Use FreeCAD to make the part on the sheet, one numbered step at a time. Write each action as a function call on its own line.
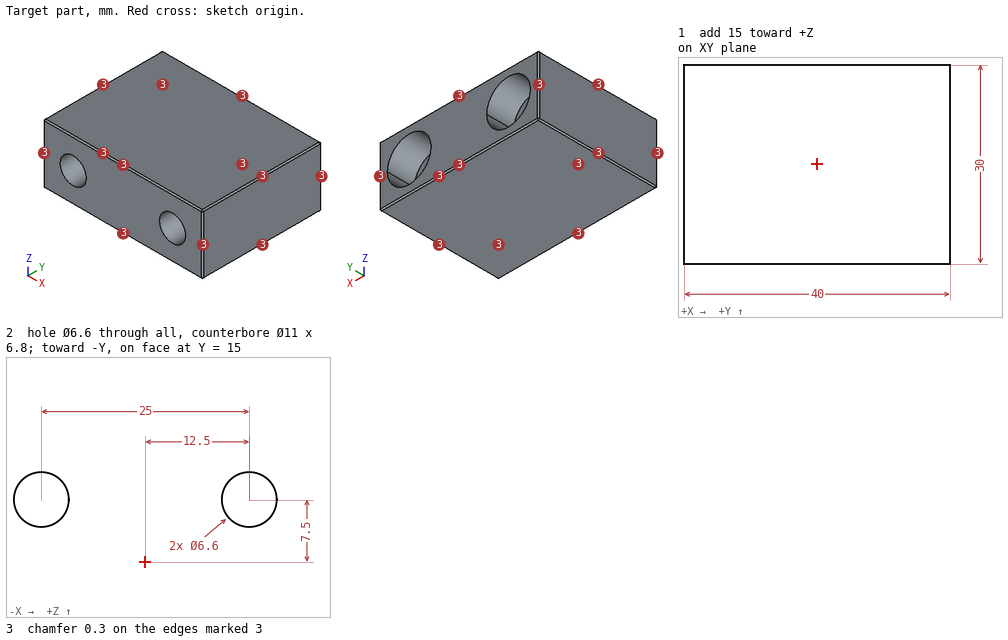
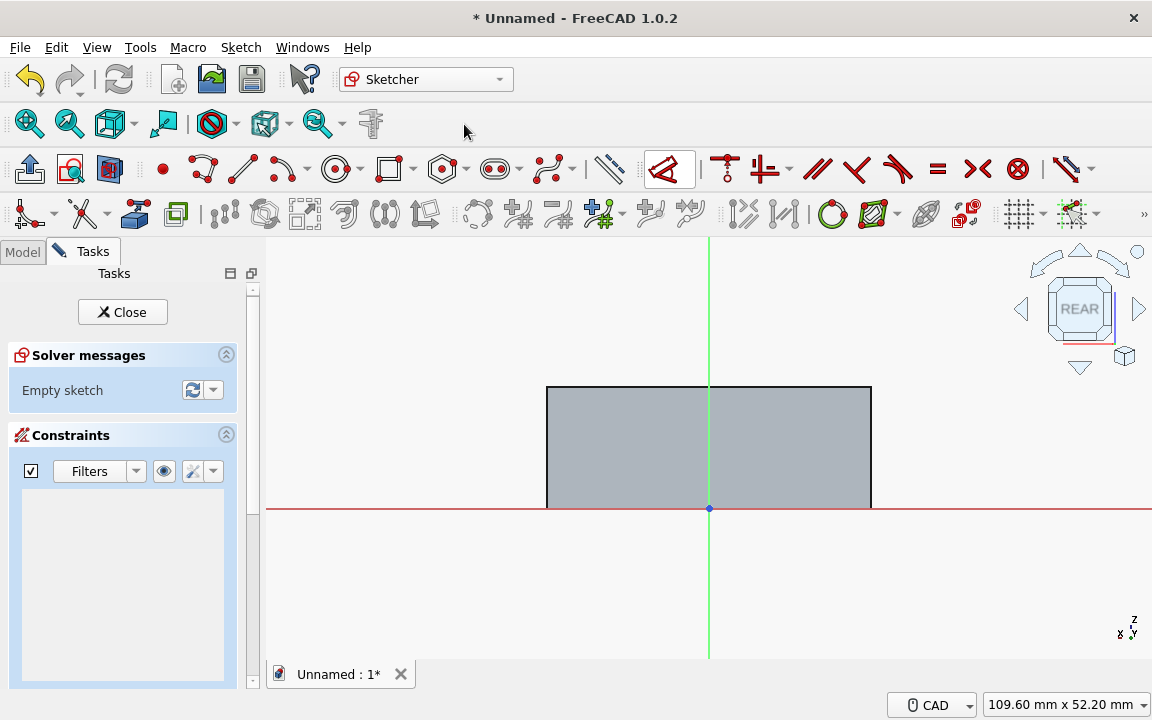
scroll(792, 486, up, 3)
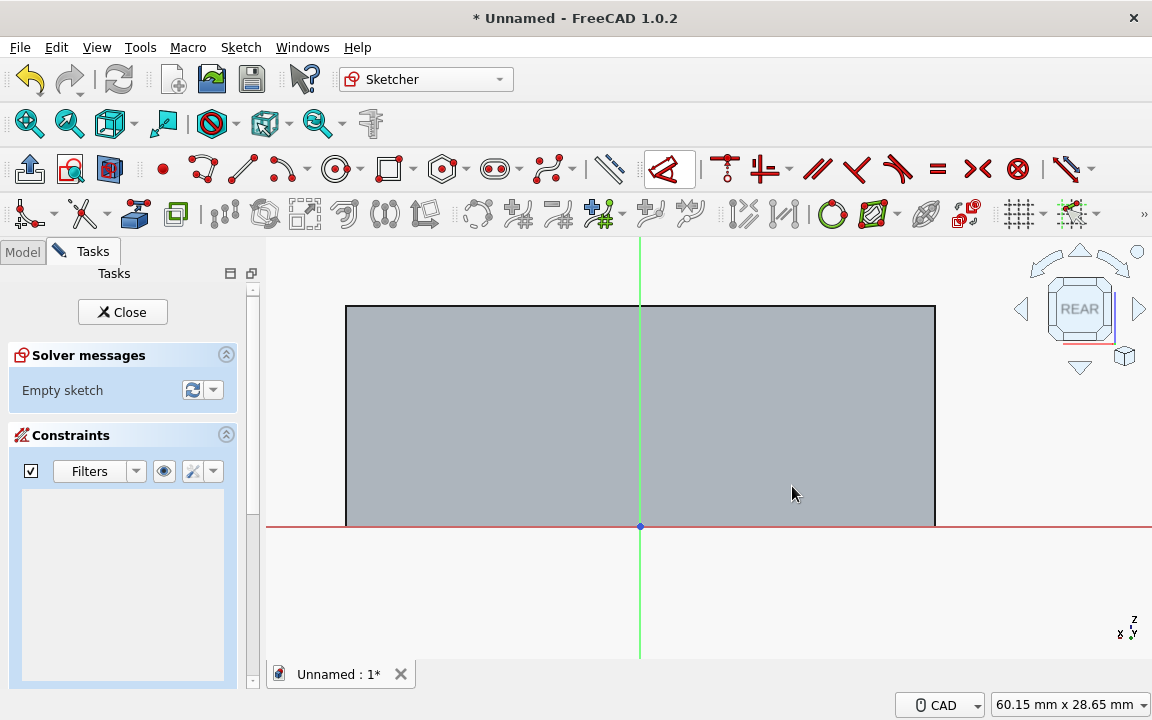
click(336, 170)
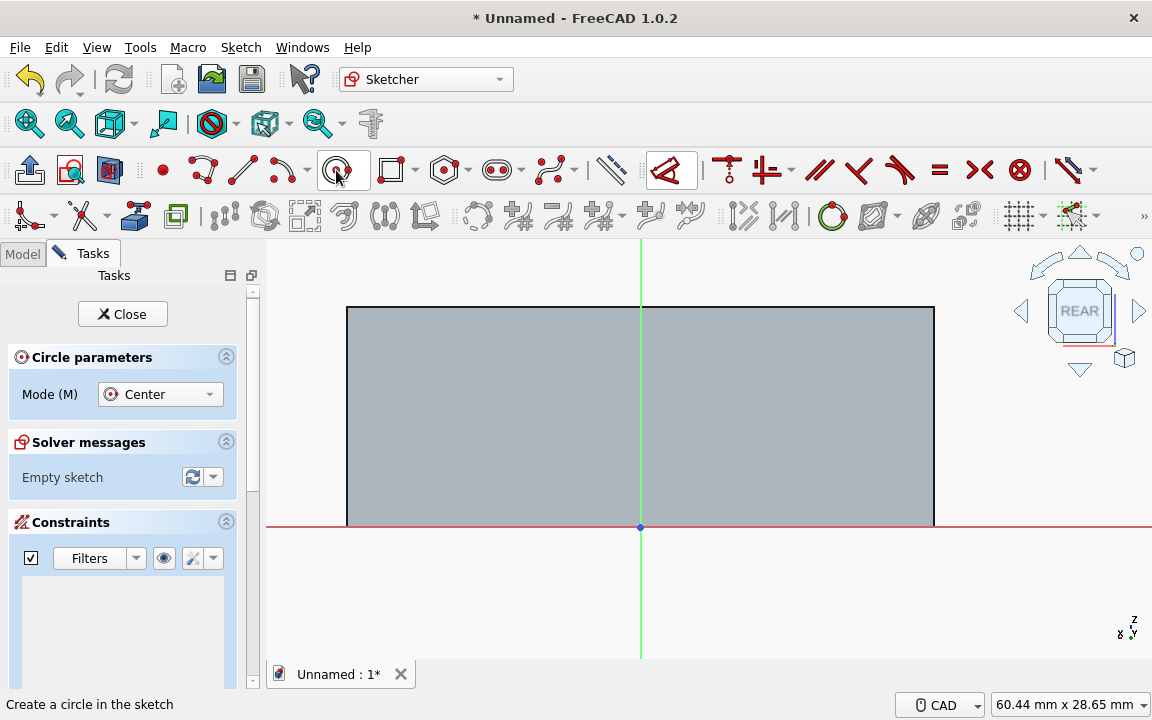
click(824, 417)
click(858, 383)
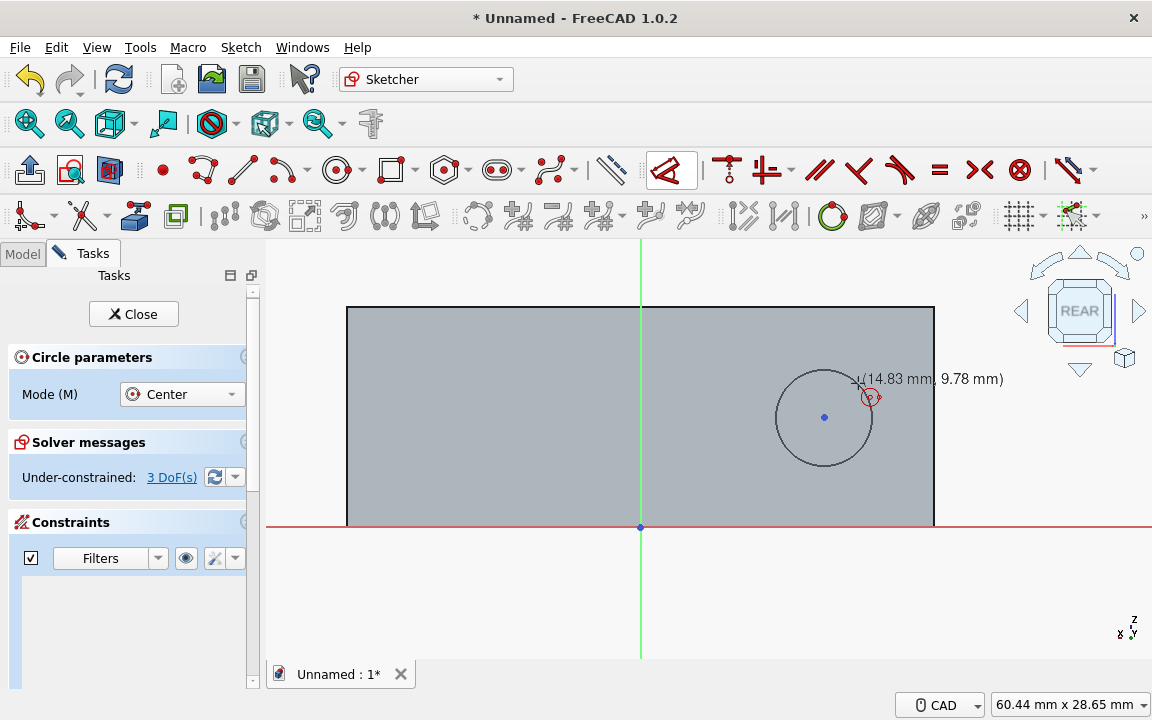
click(457, 417)
click(492, 383)
key(Escape)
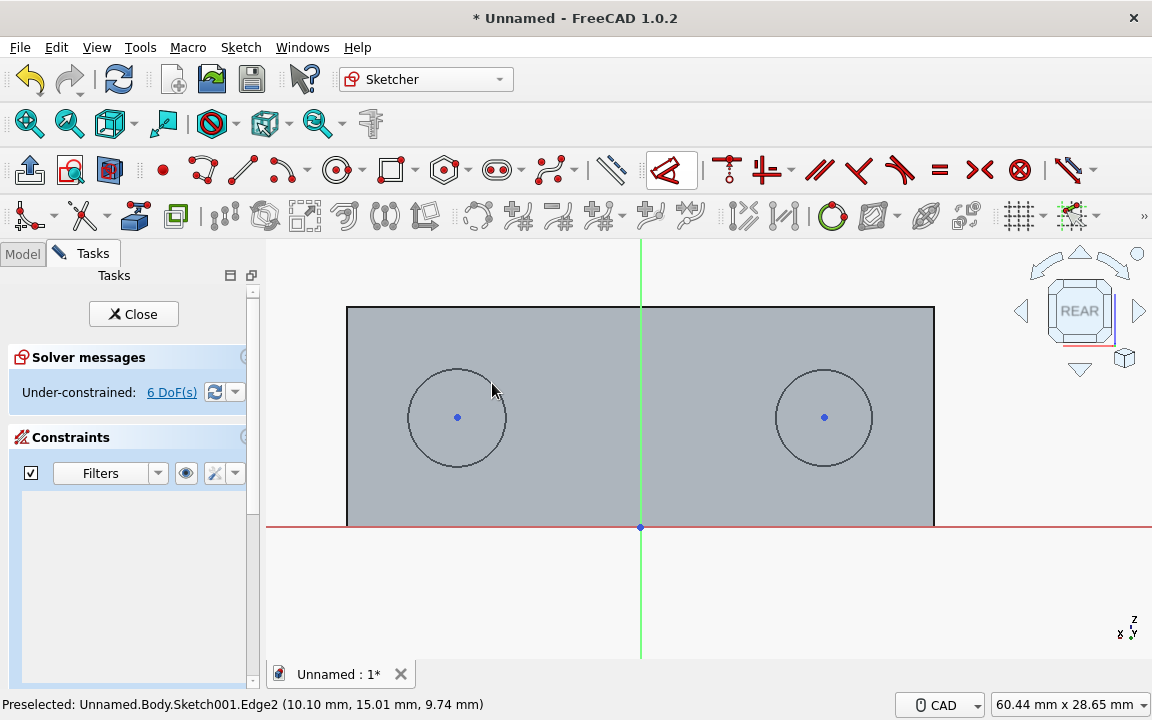
click(858, 384)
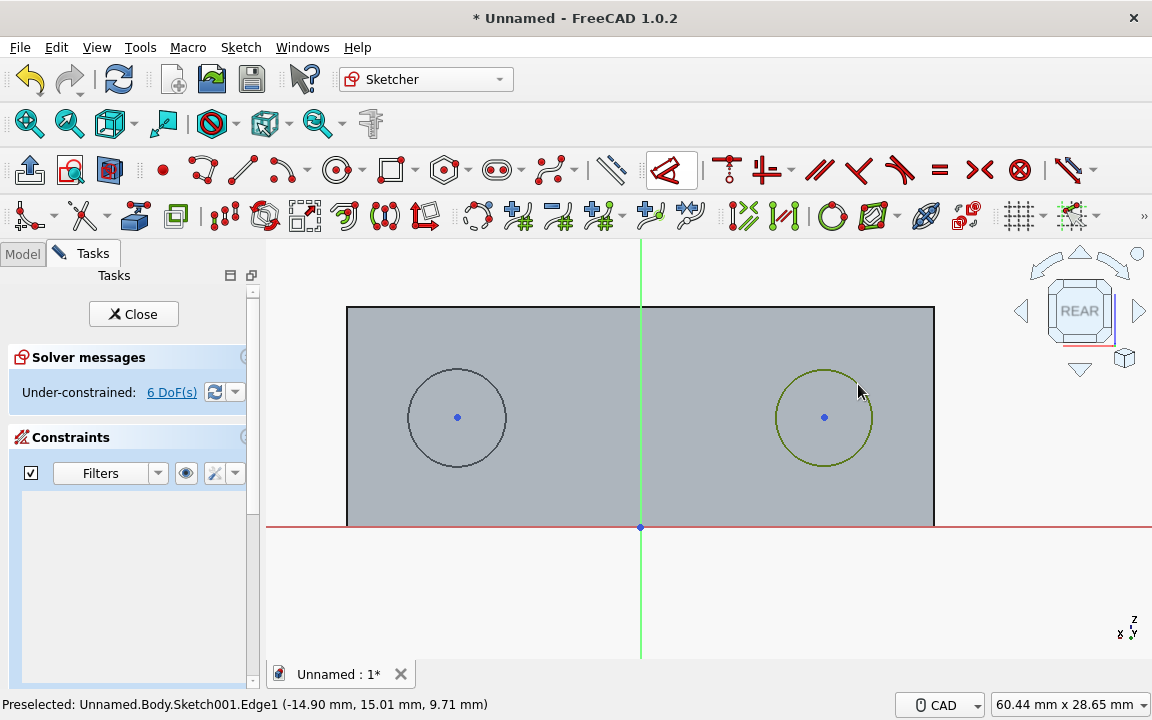
click(491, 383)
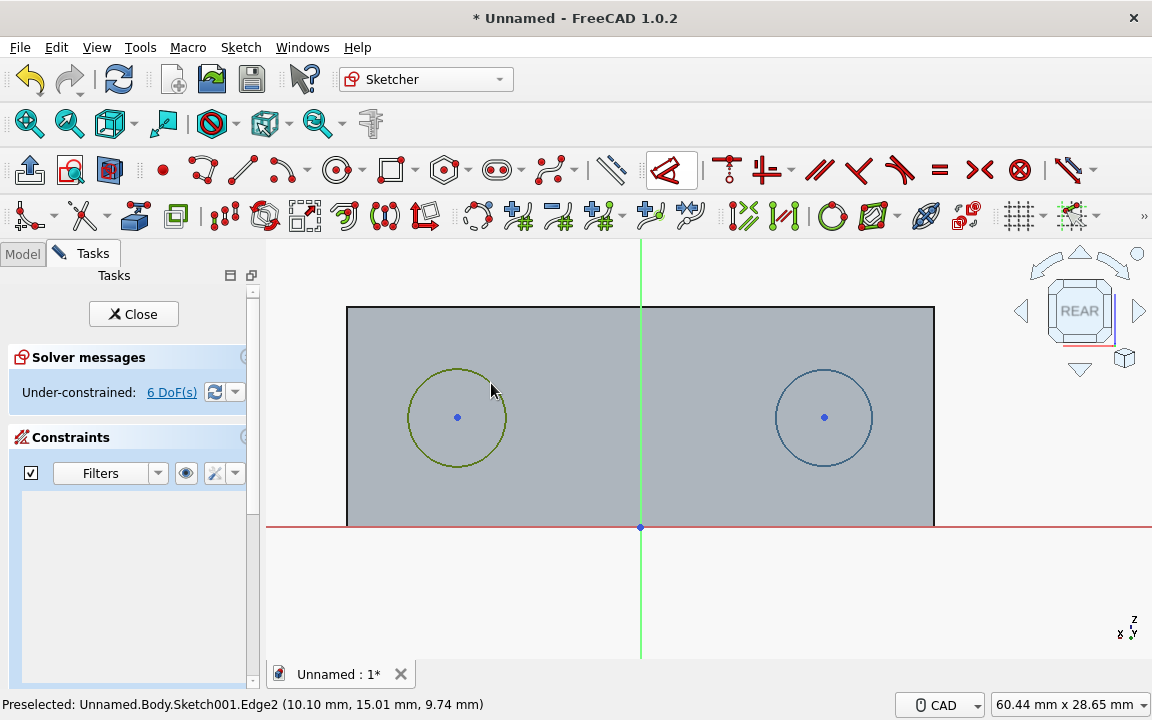
click(940, 170)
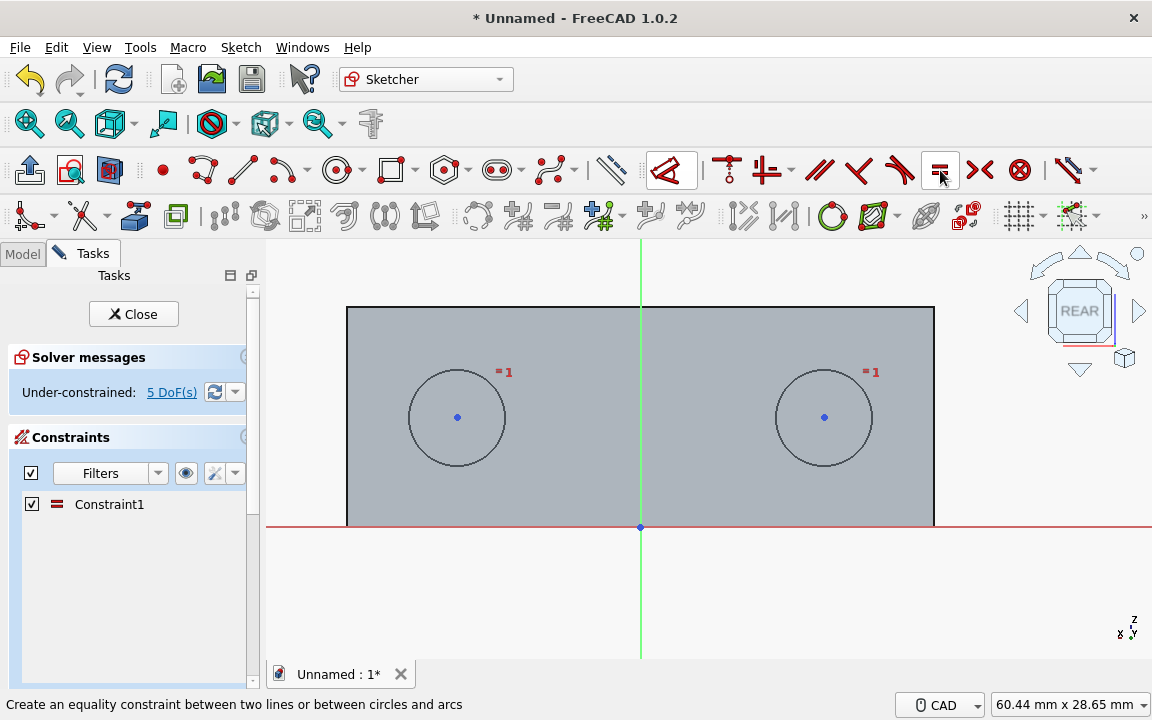
click(824, 418)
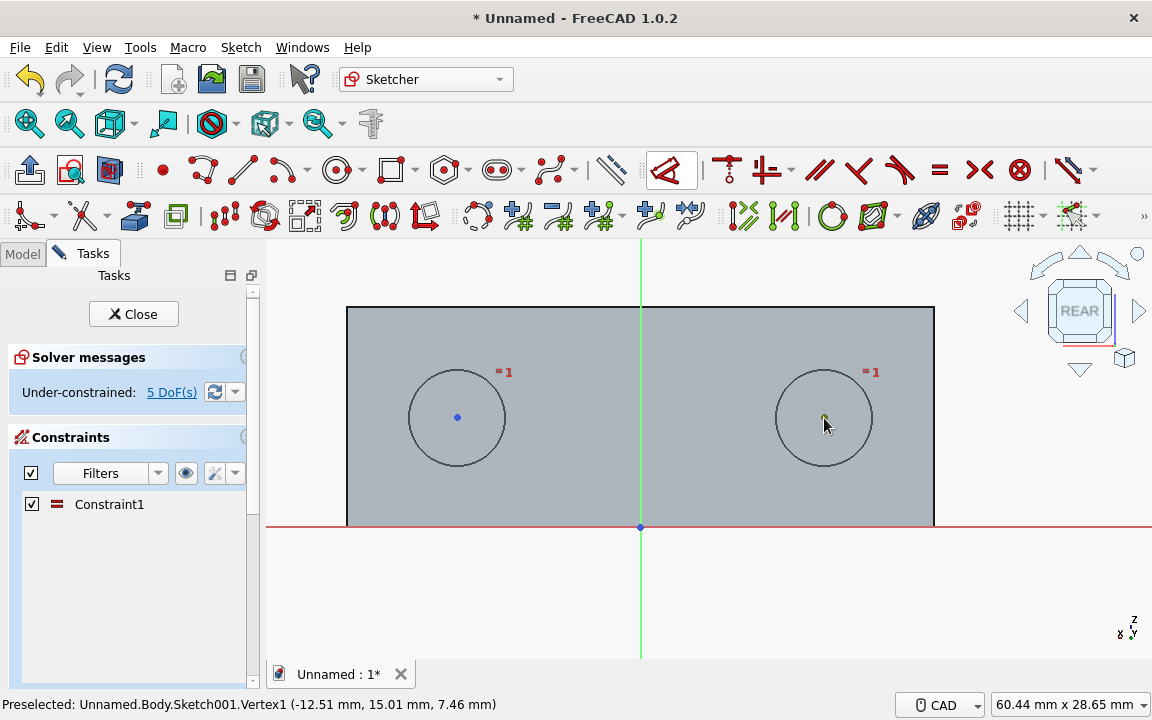
click(457, 418)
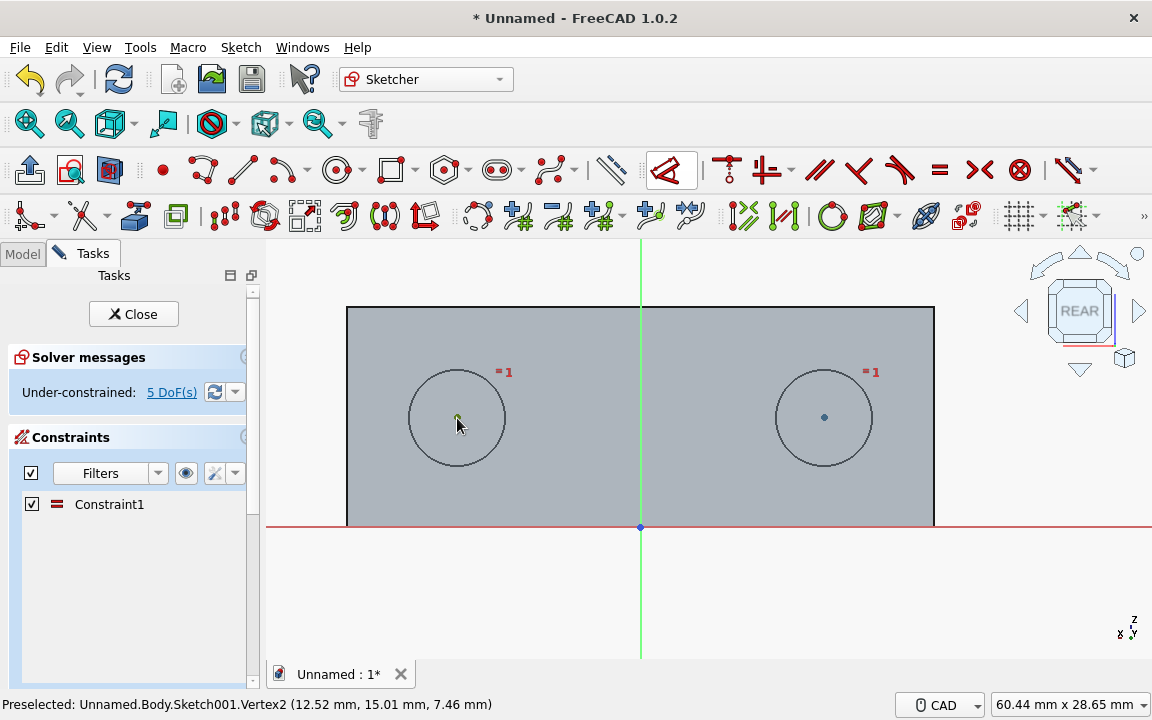
click(794, 170)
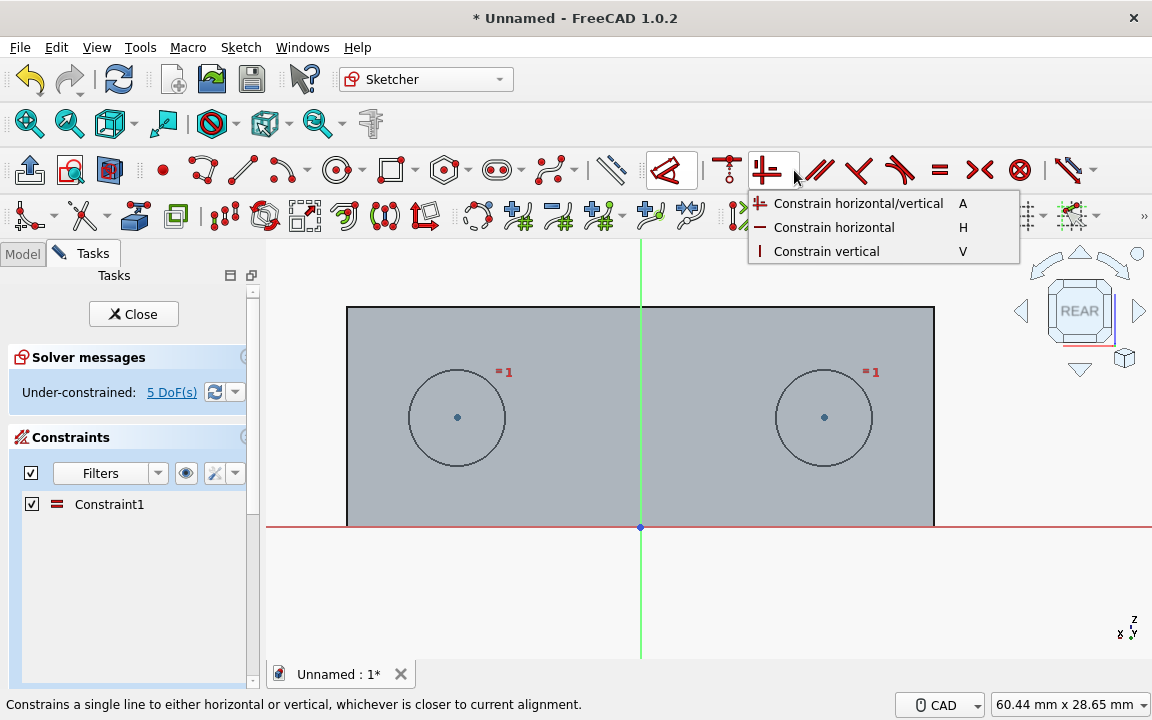
click(884, 227)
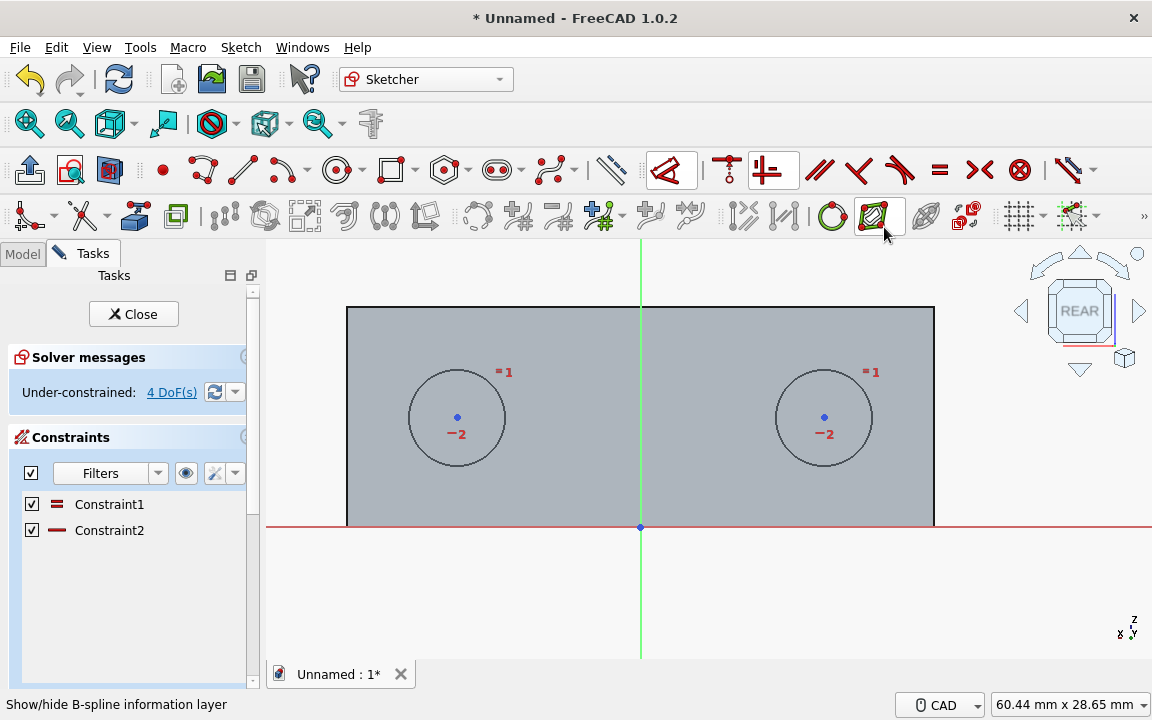
click(858, 384)